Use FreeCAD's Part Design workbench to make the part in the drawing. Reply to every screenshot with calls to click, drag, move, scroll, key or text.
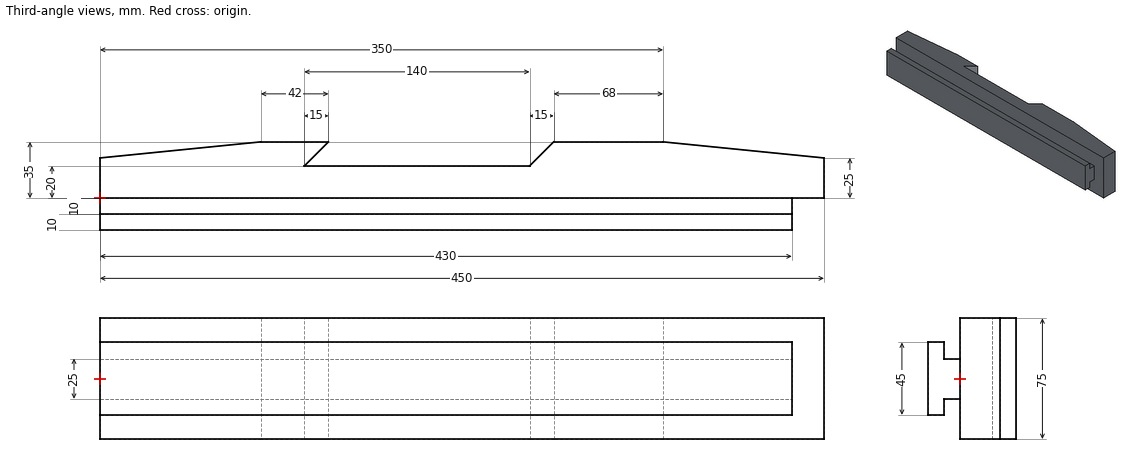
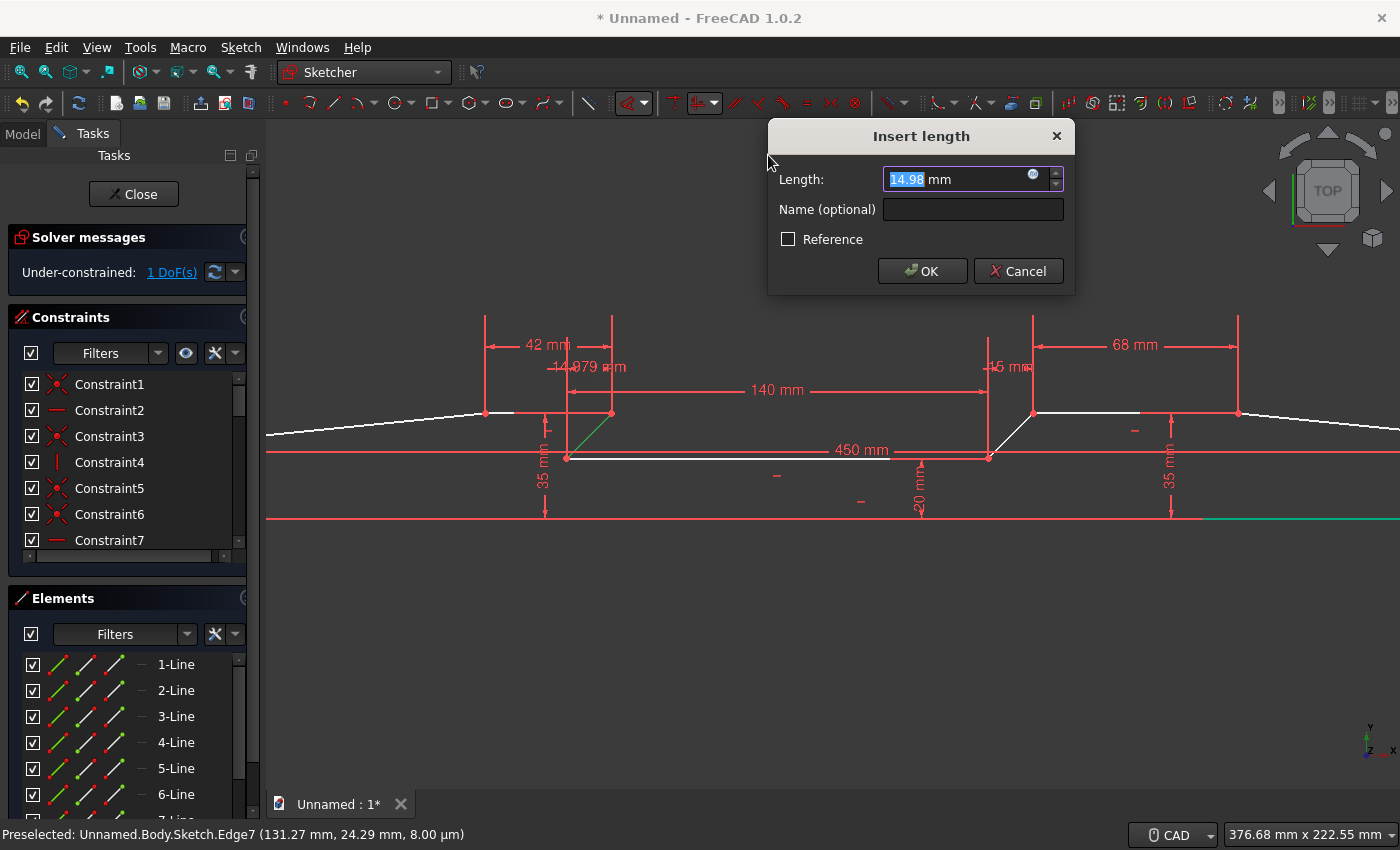
text(15)
key(Return)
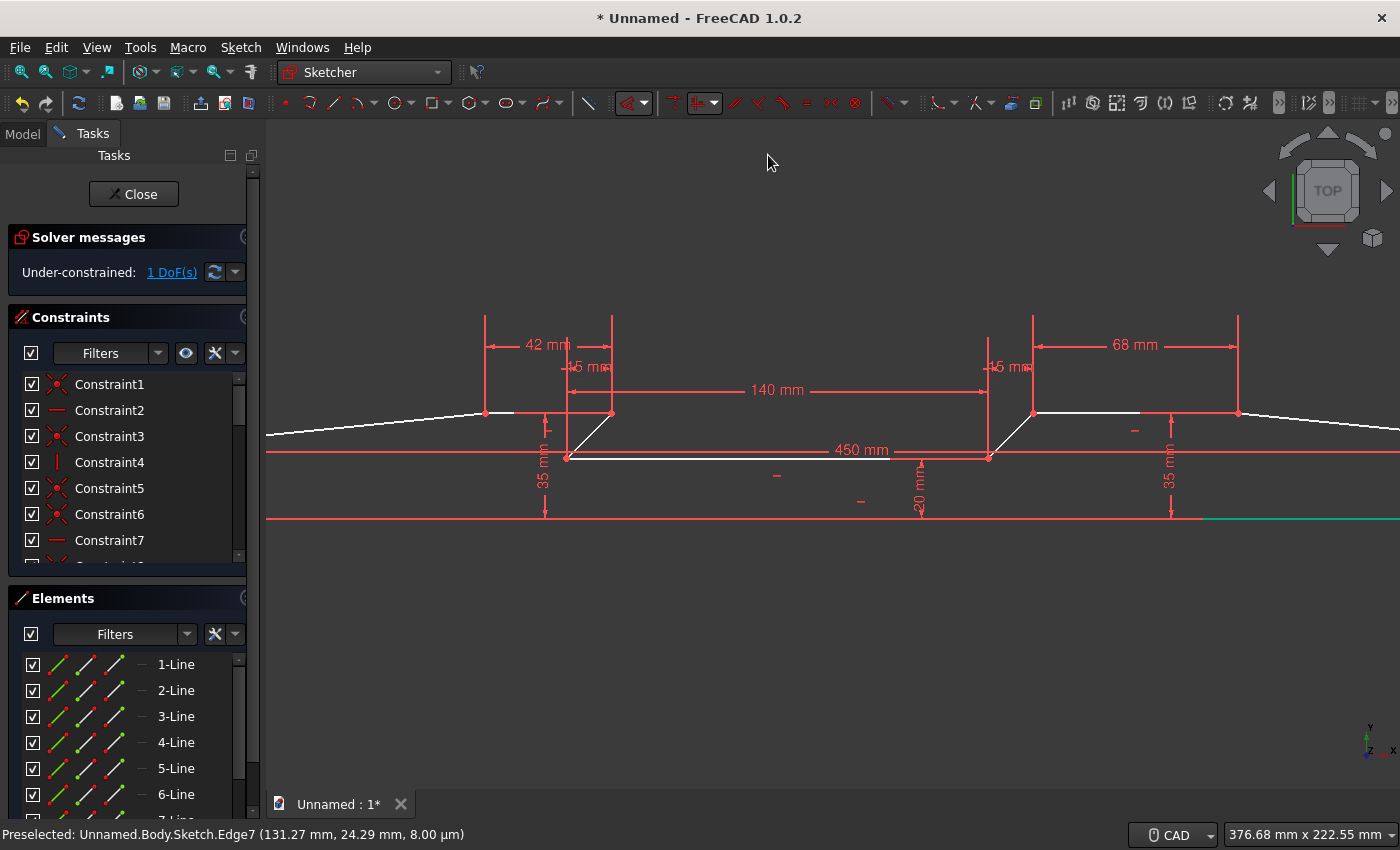
scroll(685, 444, down, 4)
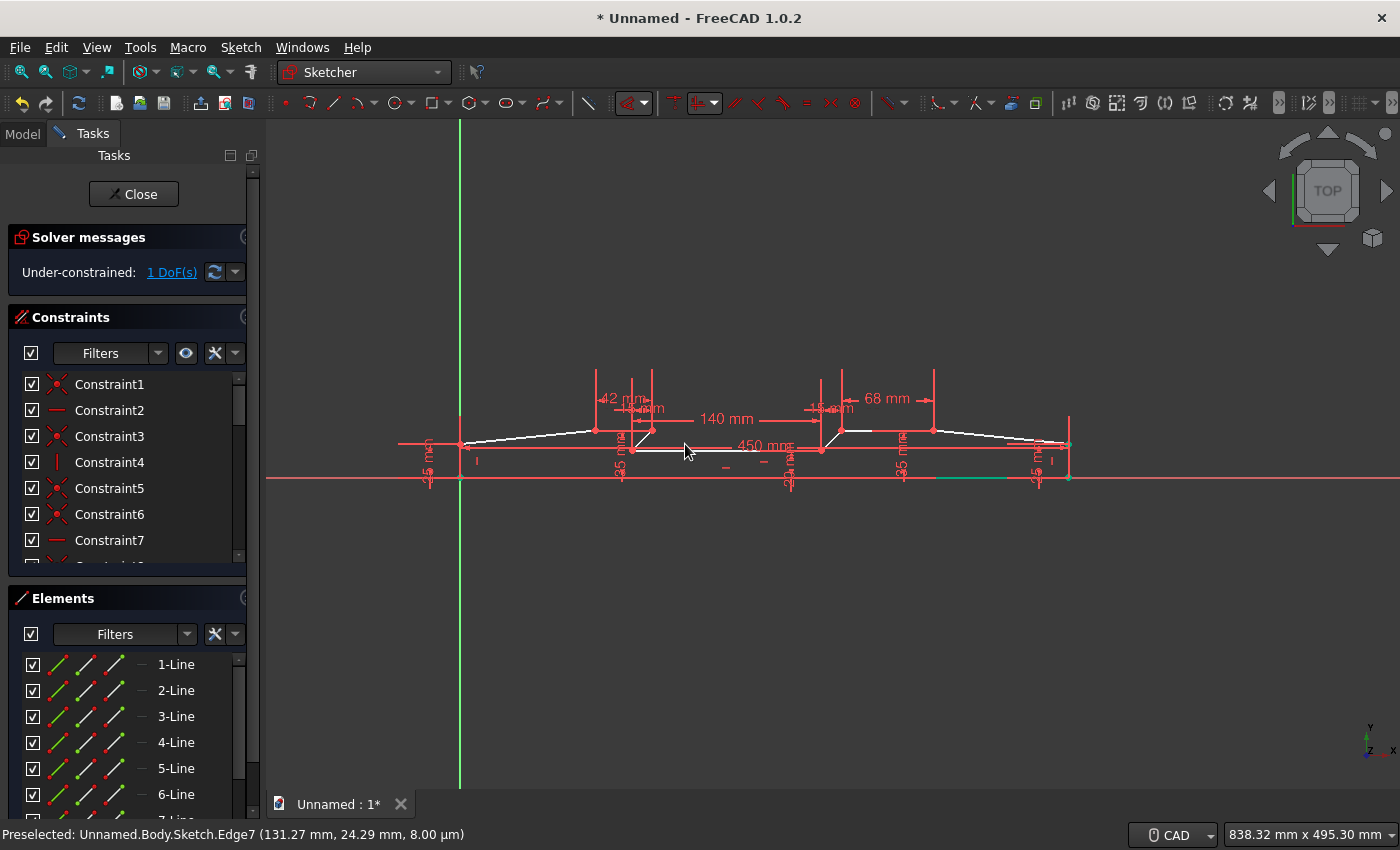
click(934, 431)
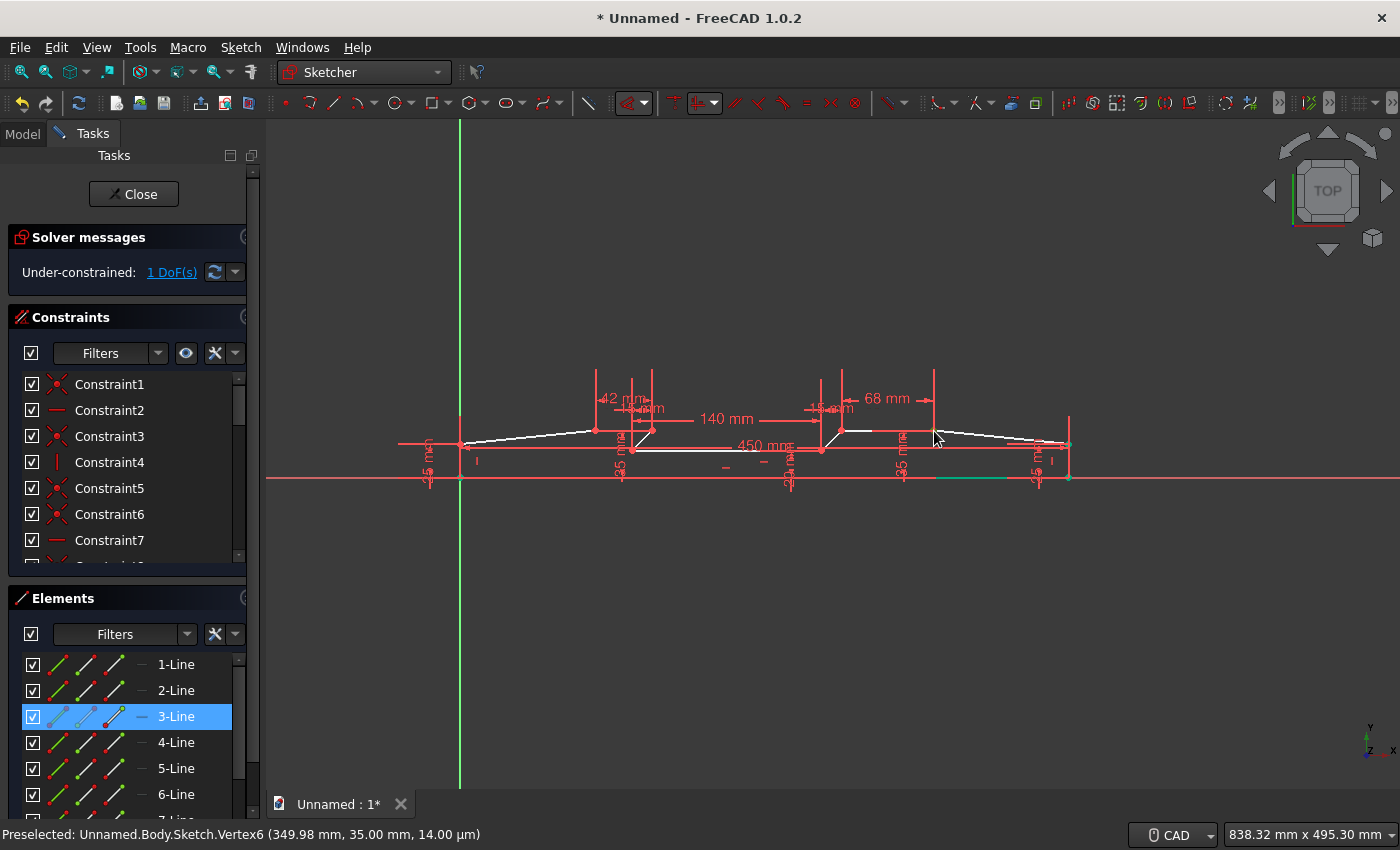
click(646, 104)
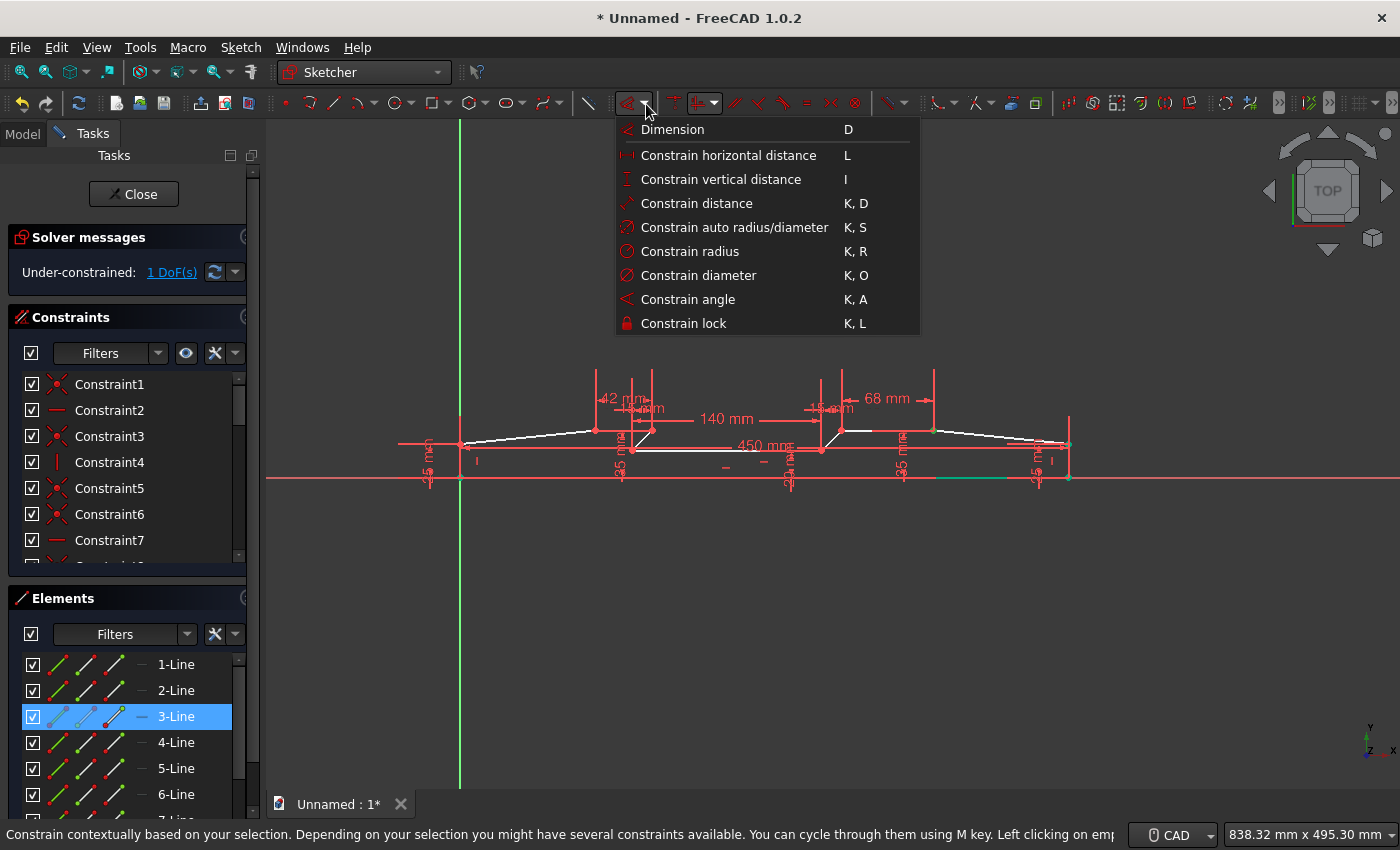
click(768, 155)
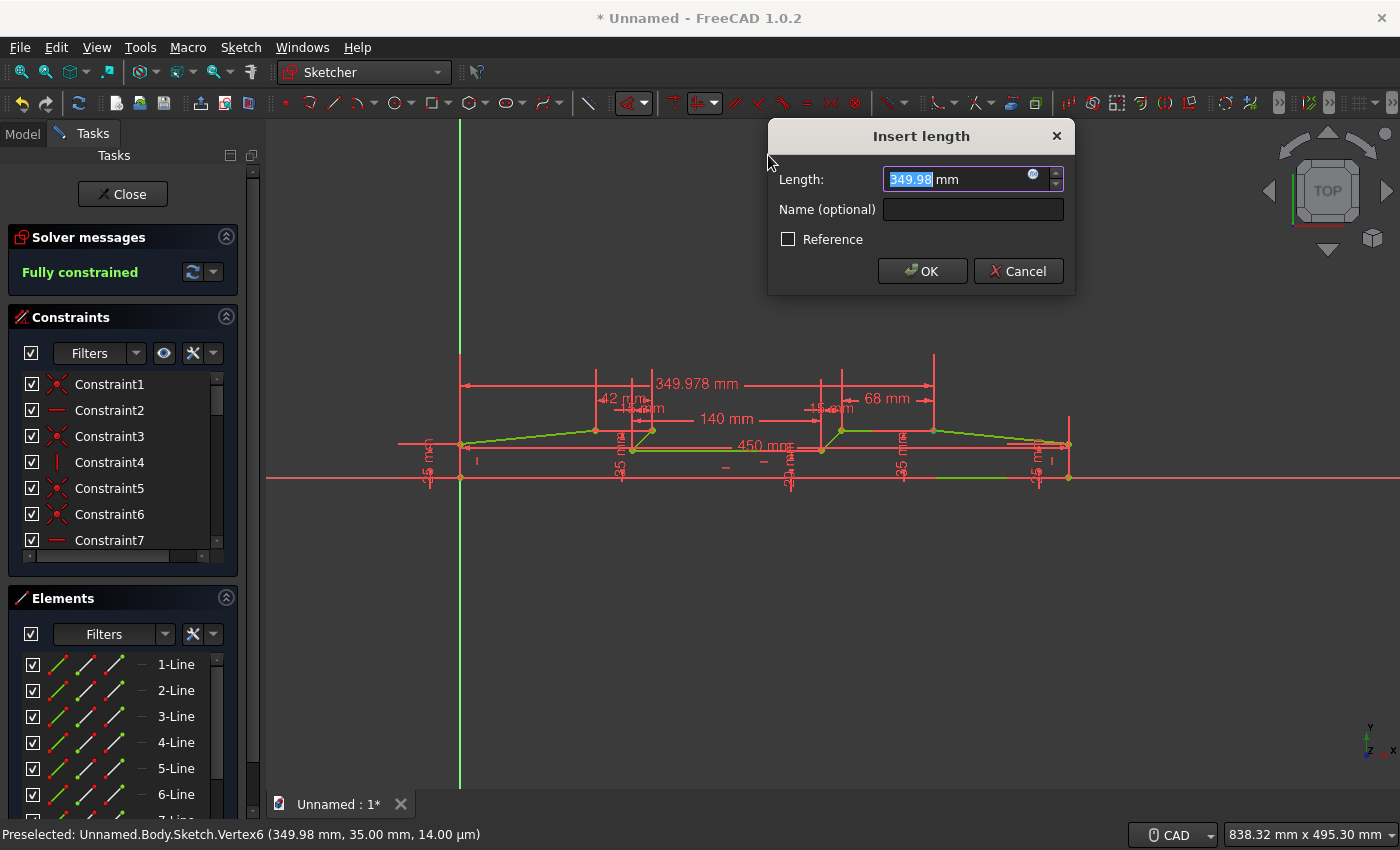
text(350)
key(Return)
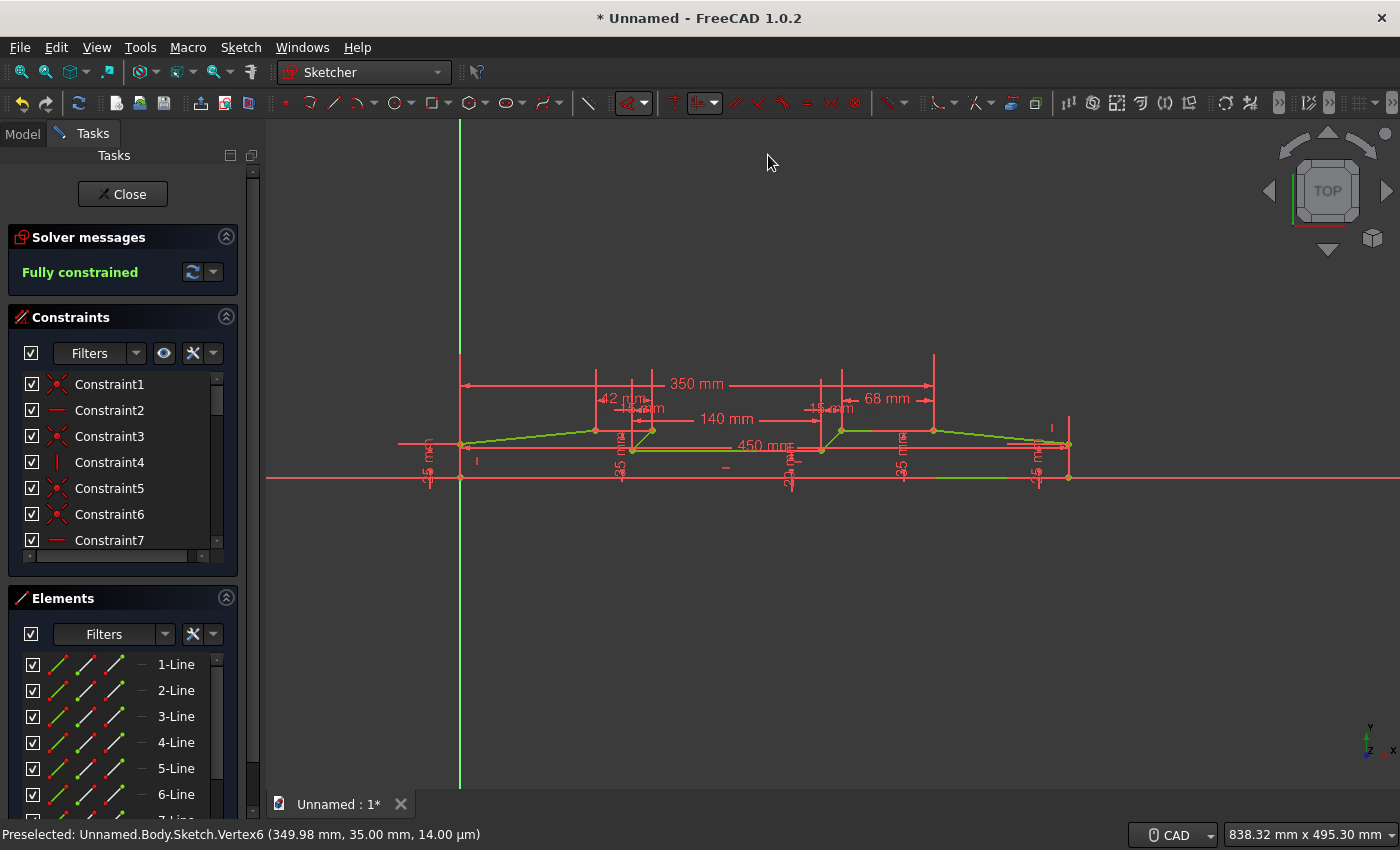
click(123, 194)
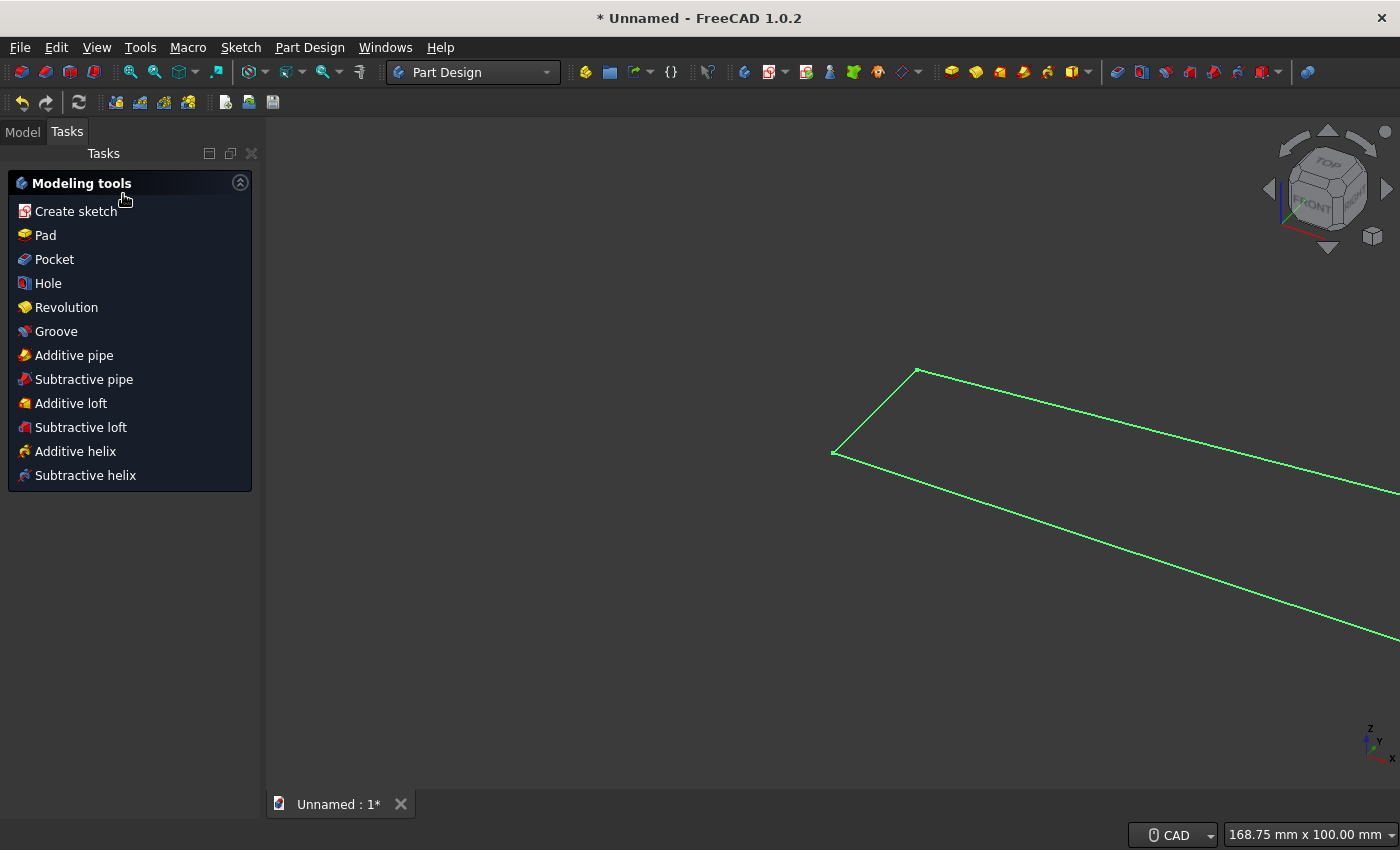
click(952, 72)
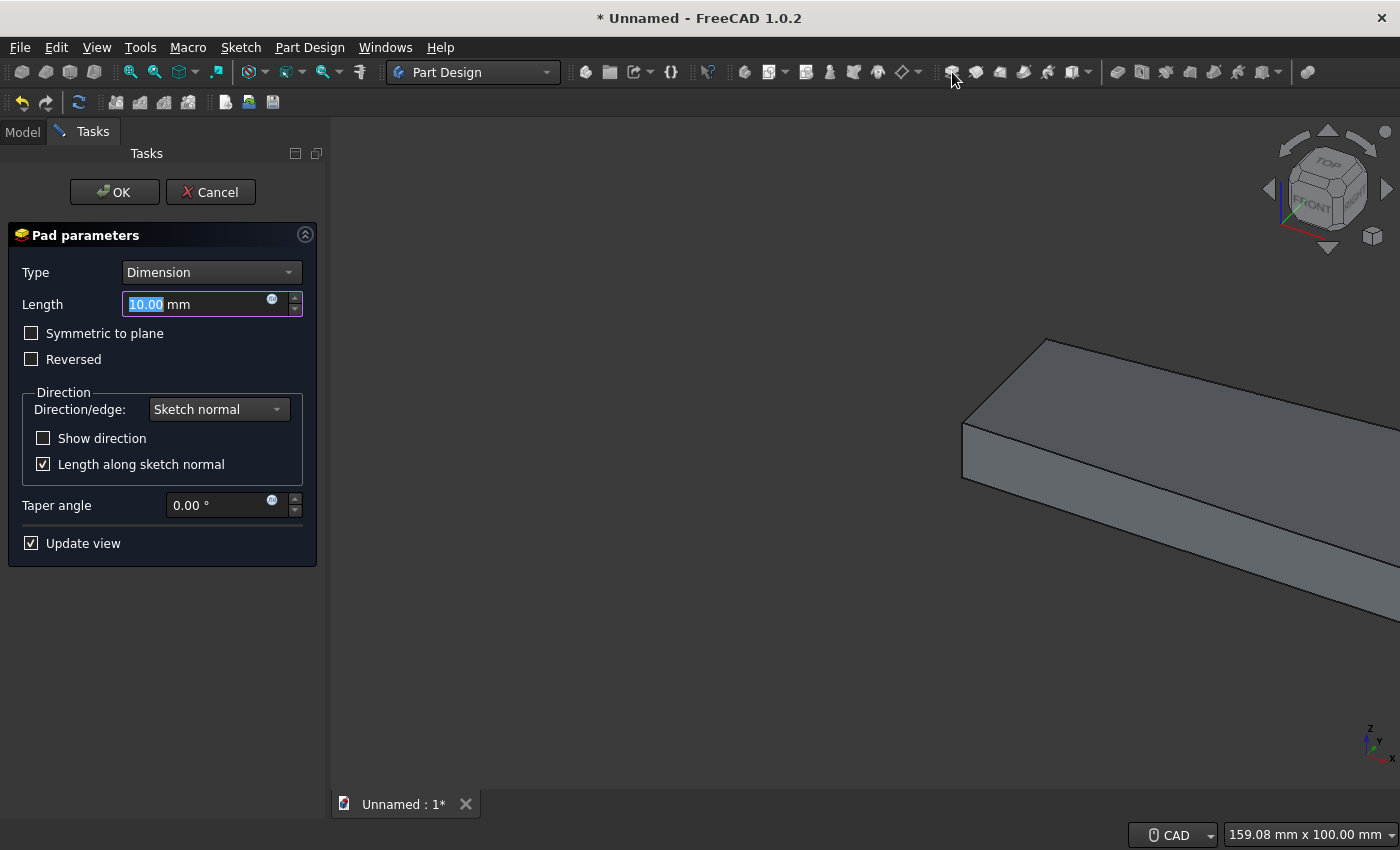
text(75)
key(Tab)